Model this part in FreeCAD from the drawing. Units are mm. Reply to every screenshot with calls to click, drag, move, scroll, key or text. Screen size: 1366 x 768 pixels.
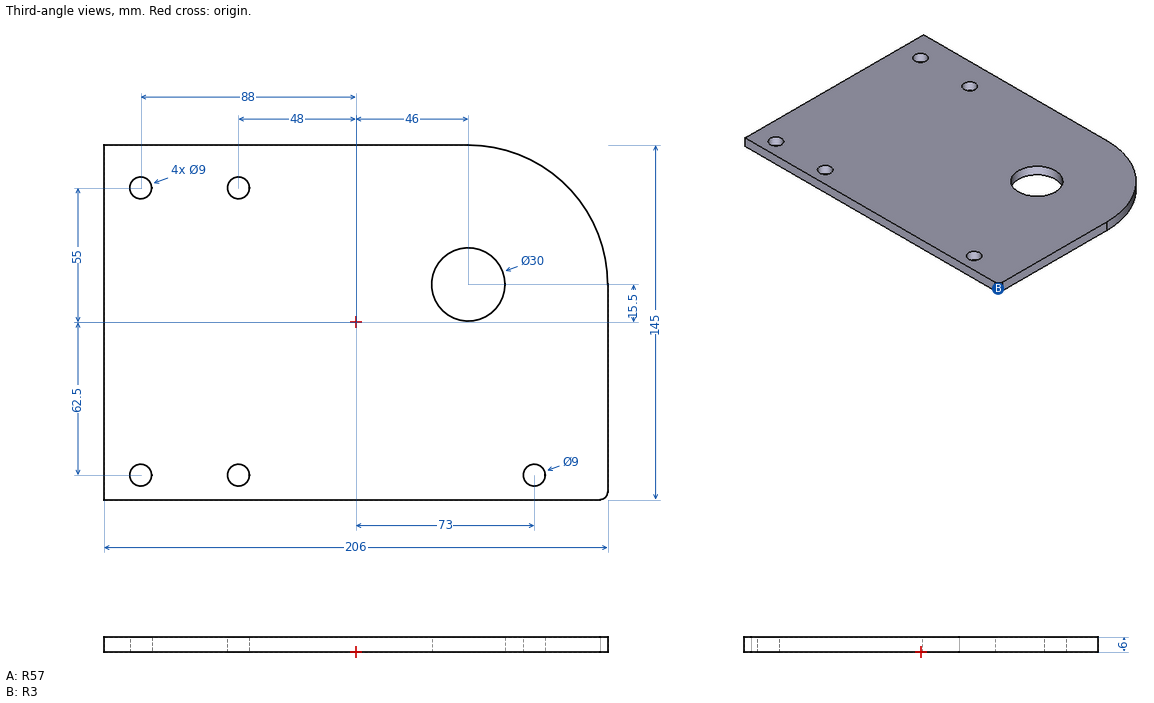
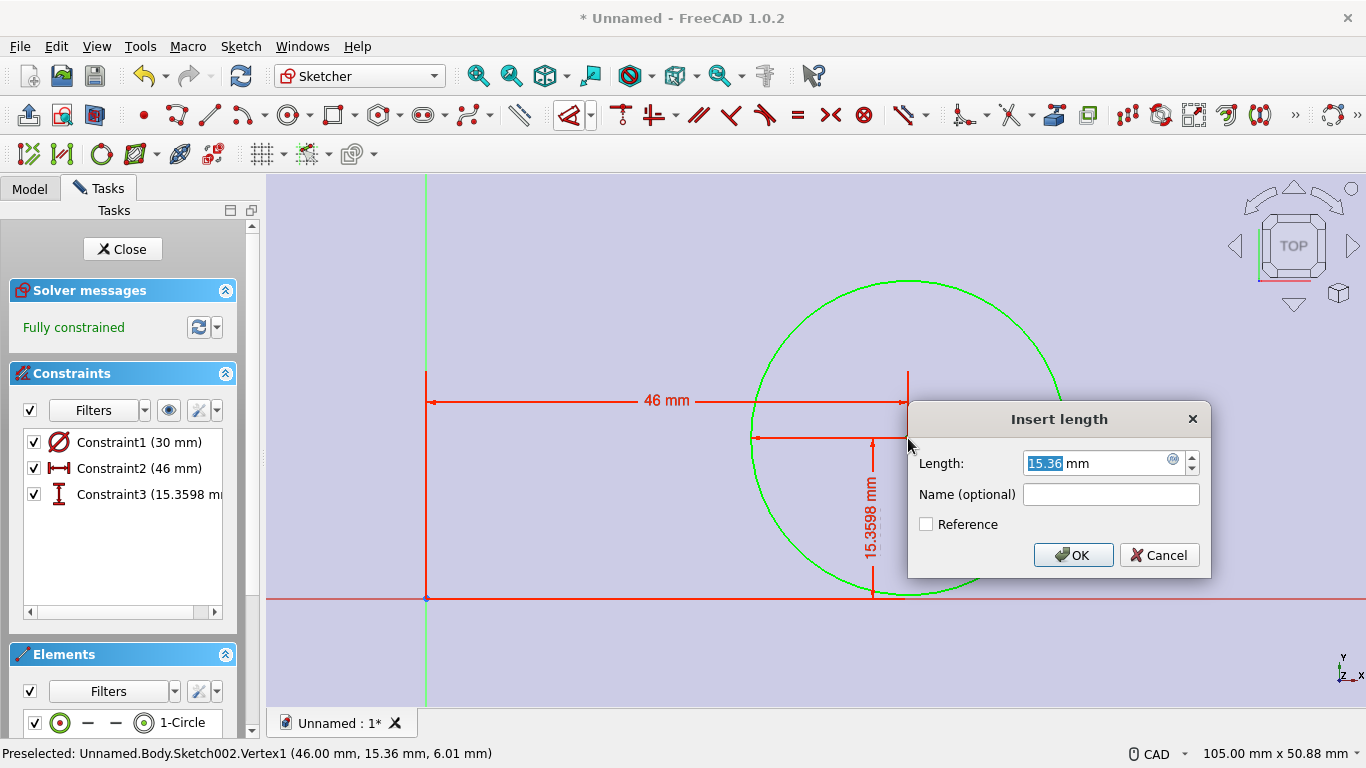
text(15.5)
key(Return)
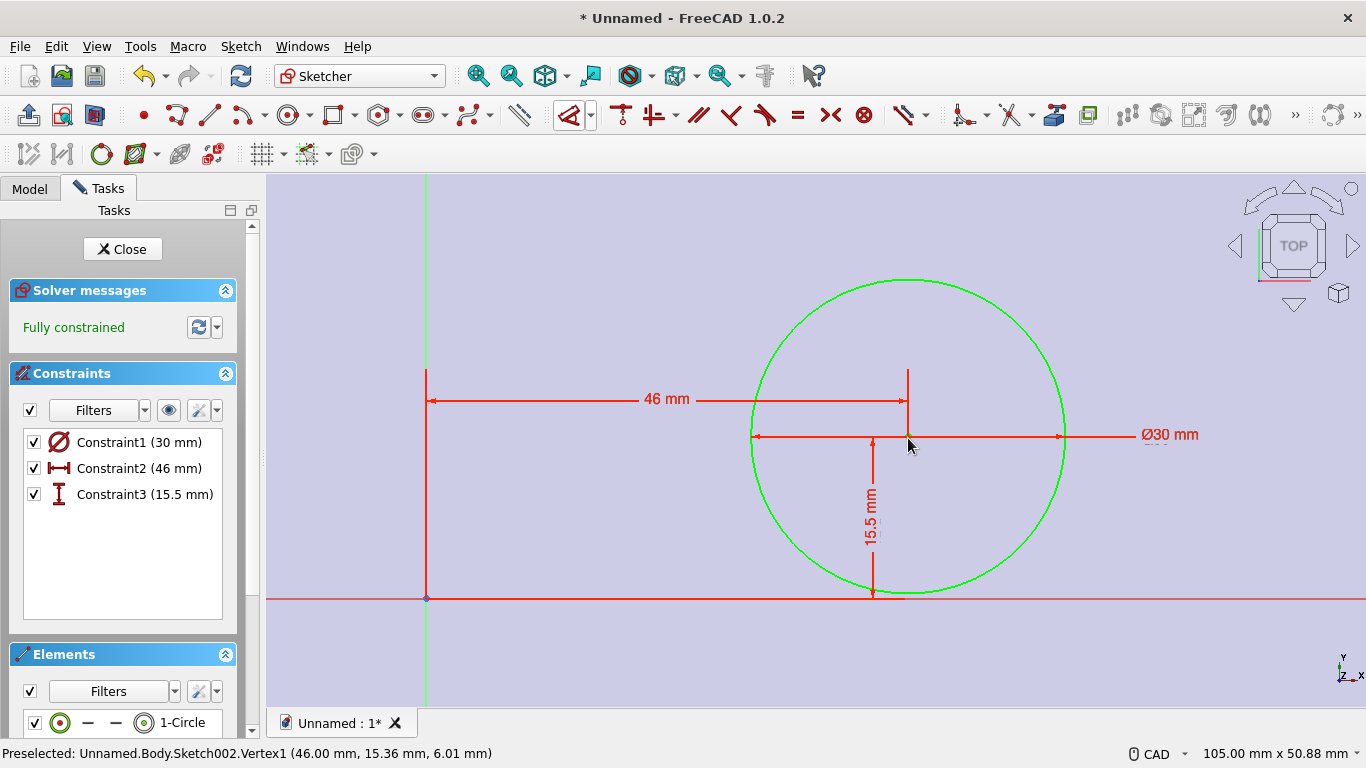
click(123, 249)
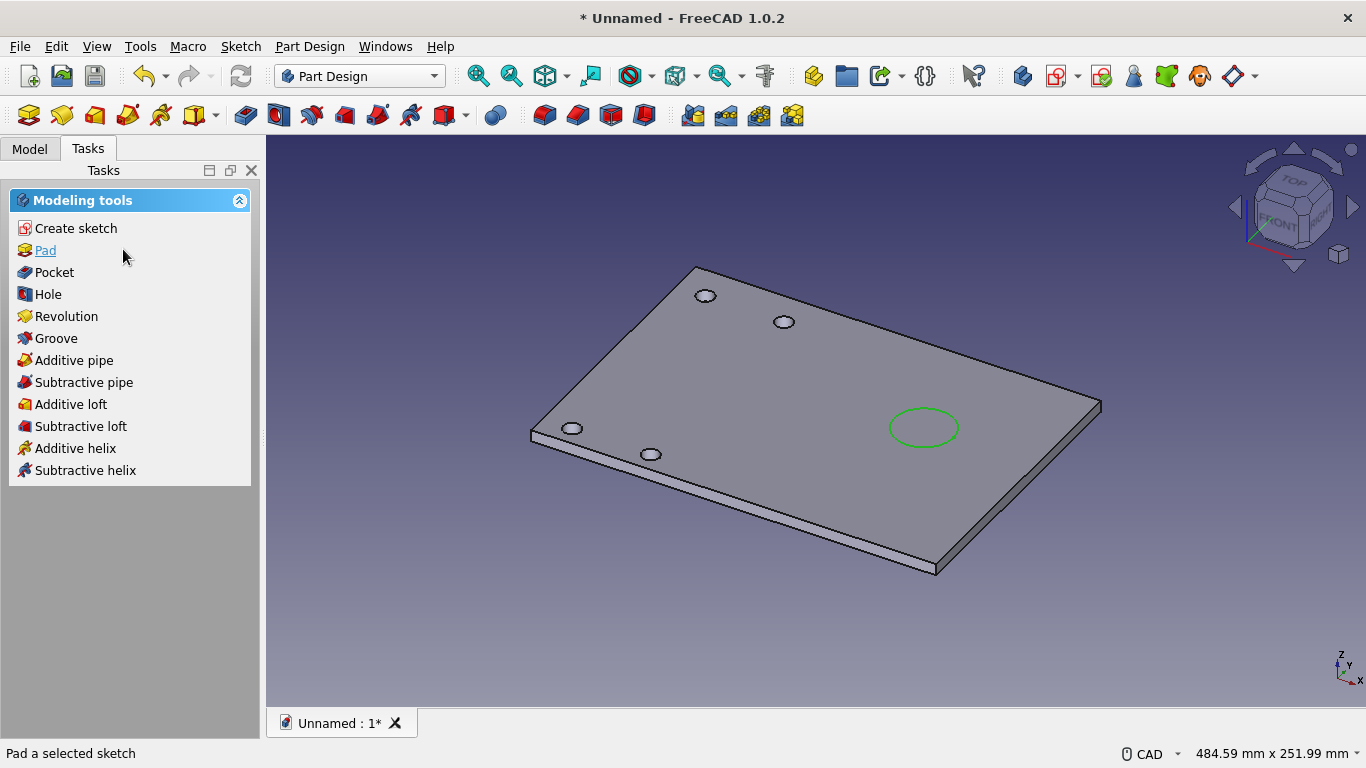
click(246, 116)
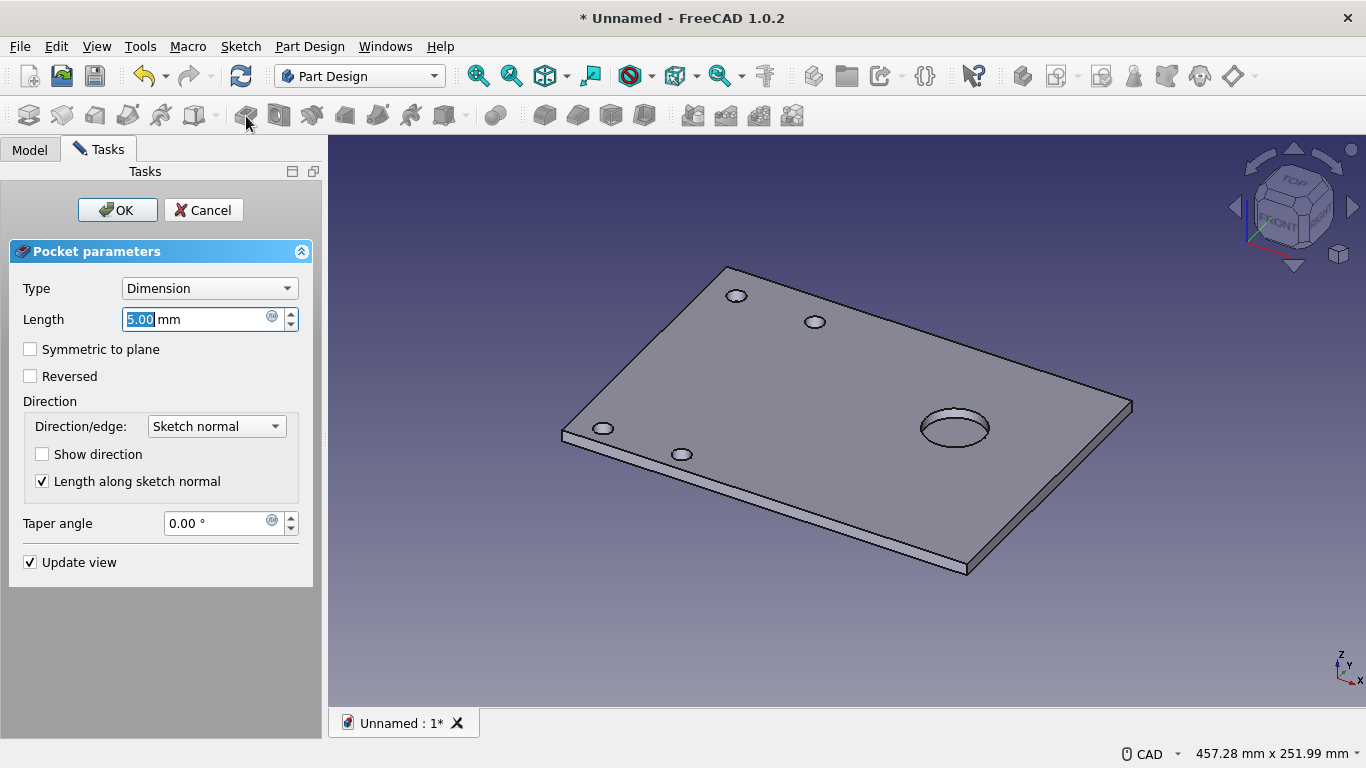
click(210, 288)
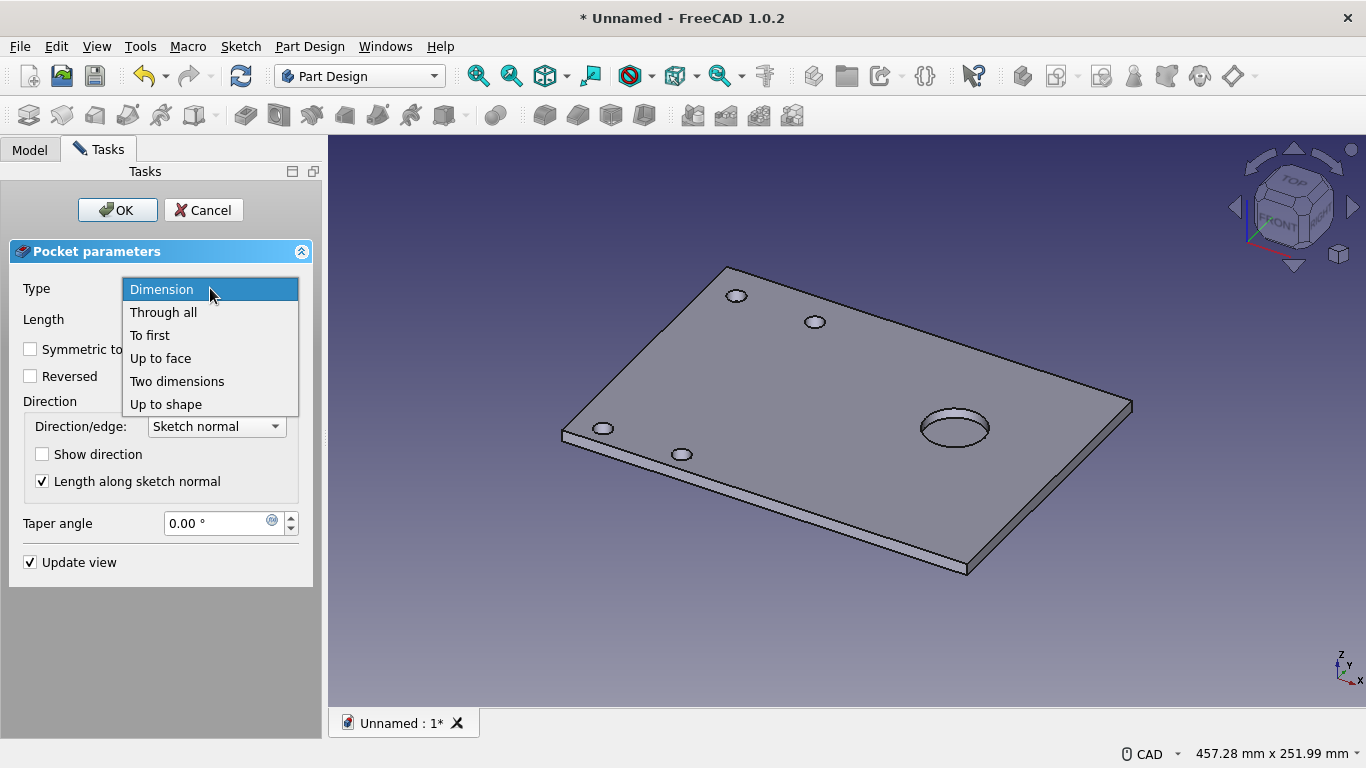
click(208, 312)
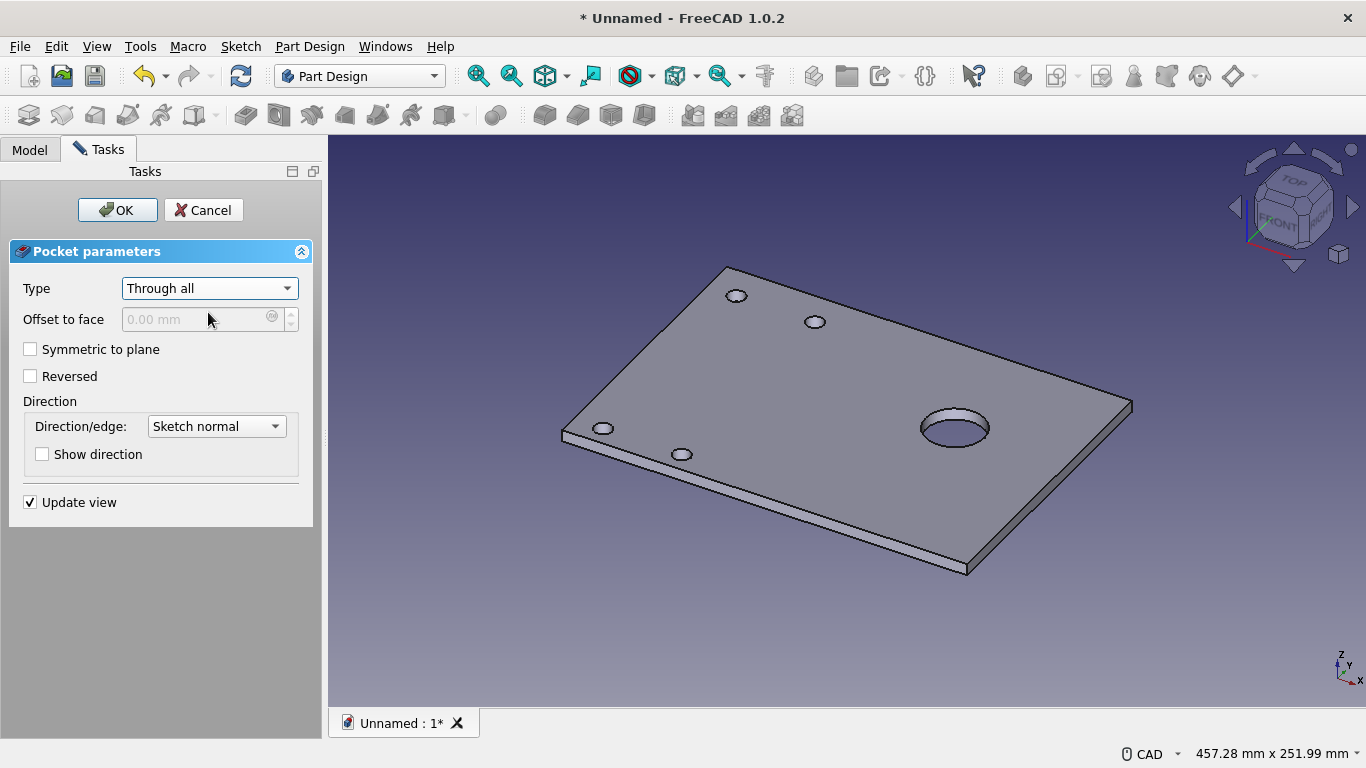
click(118, 210)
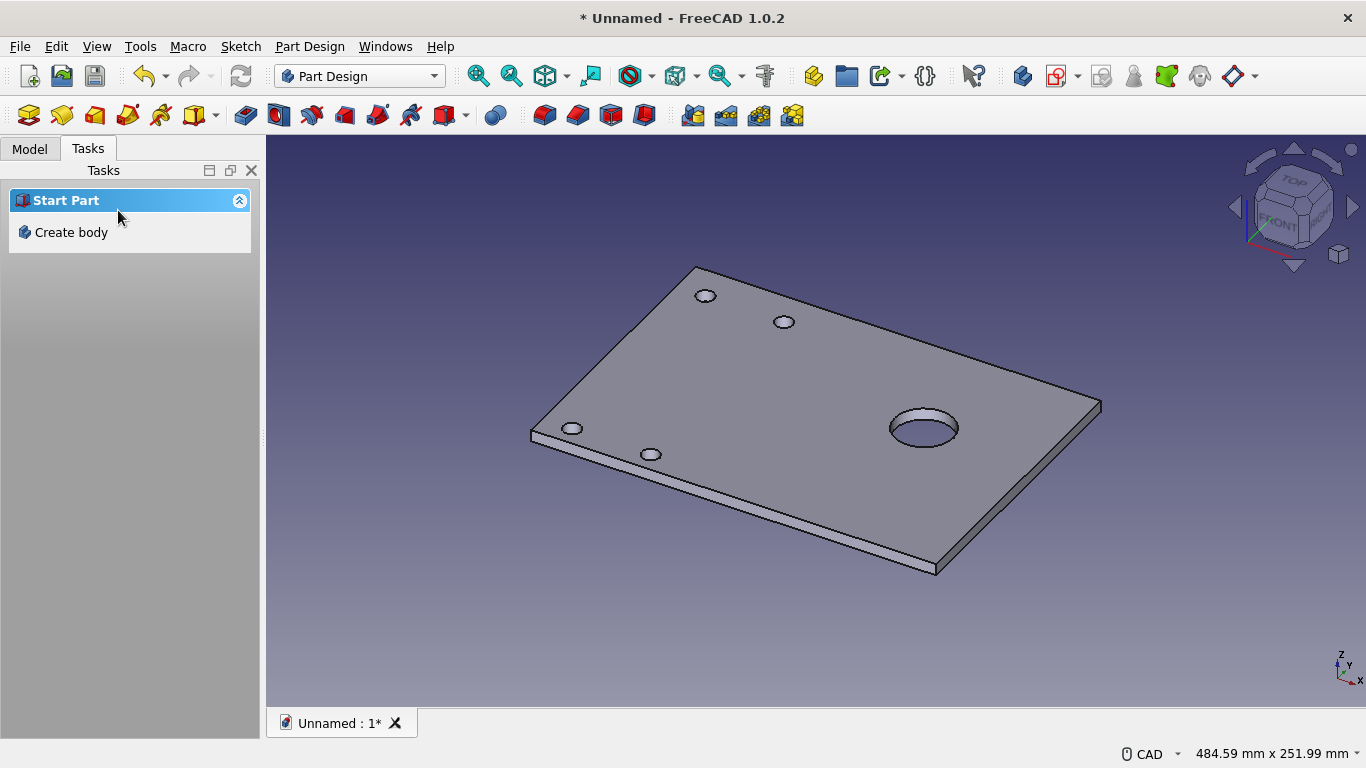
scroll(1101, 405, up, 6)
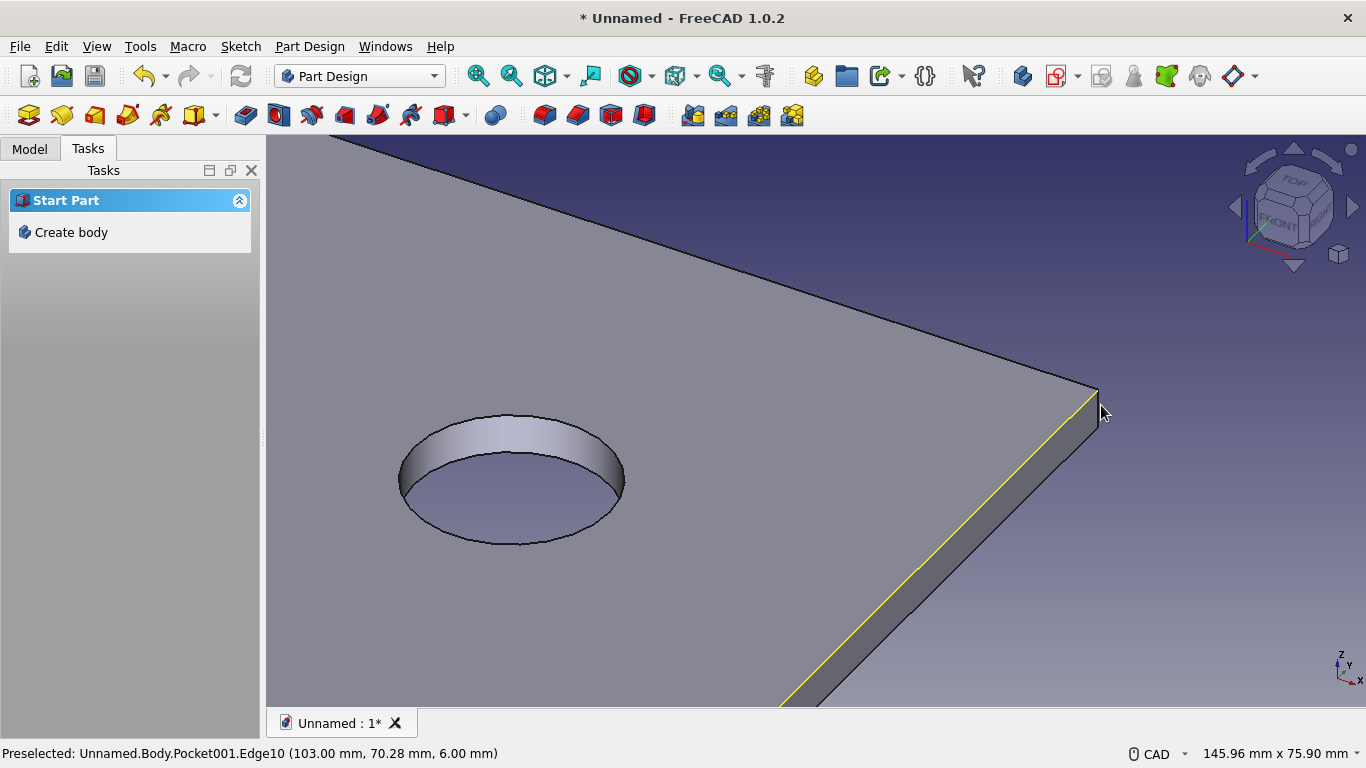
click(479, 76)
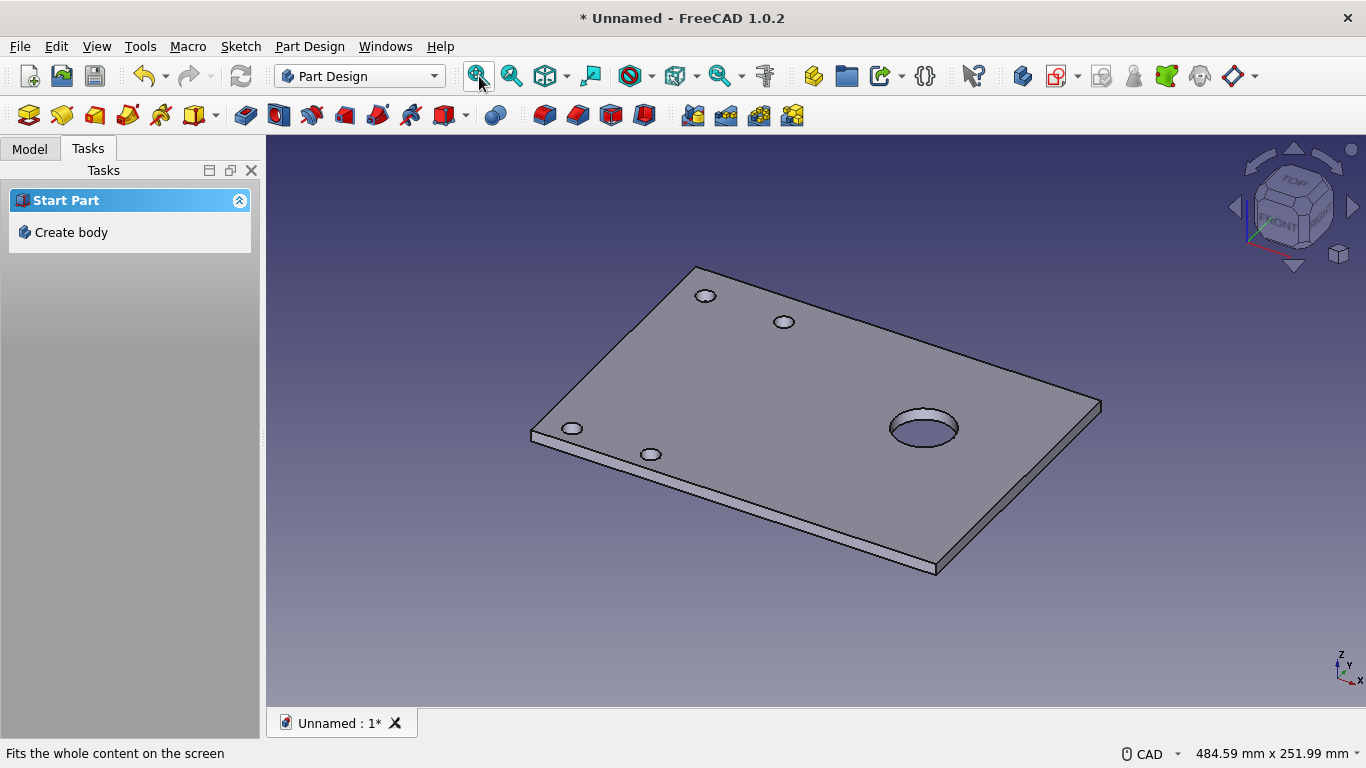
key(0)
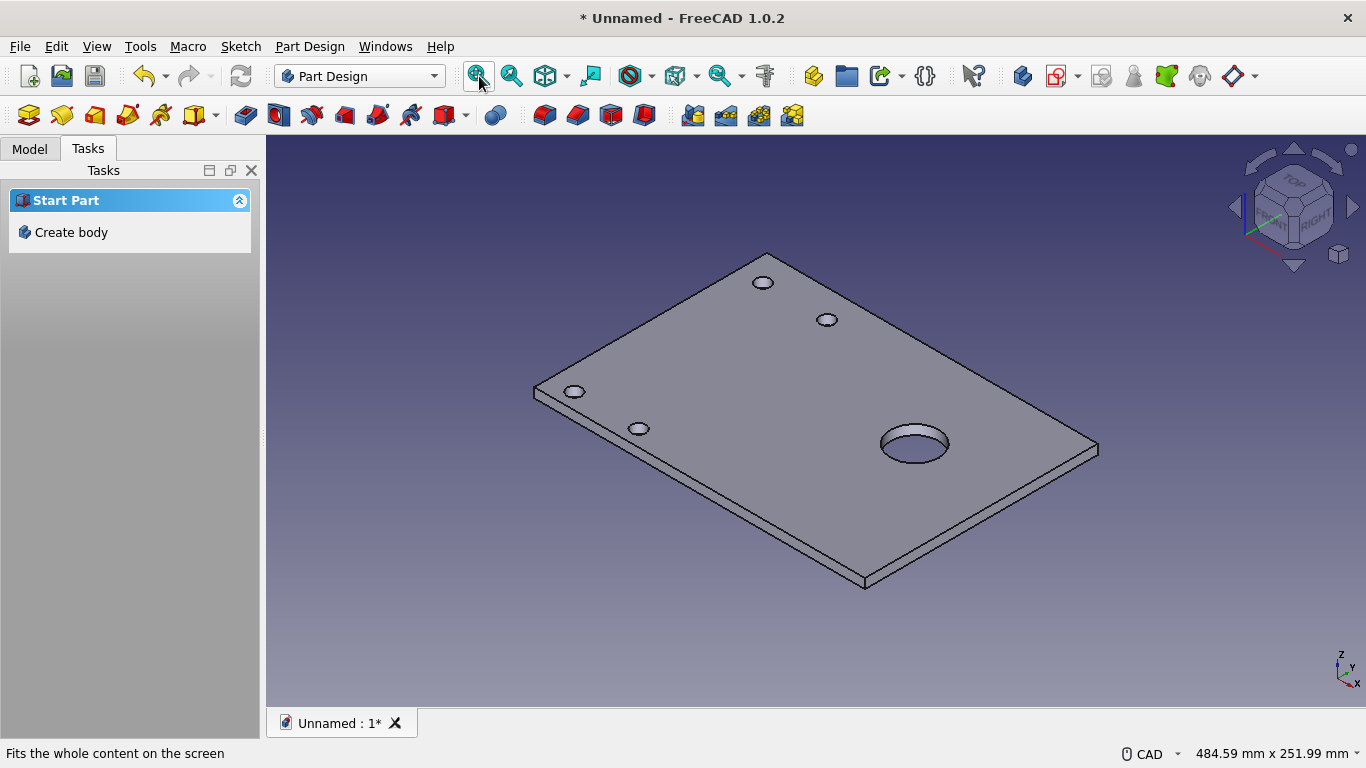
scroll(1098, 448, up, 6)